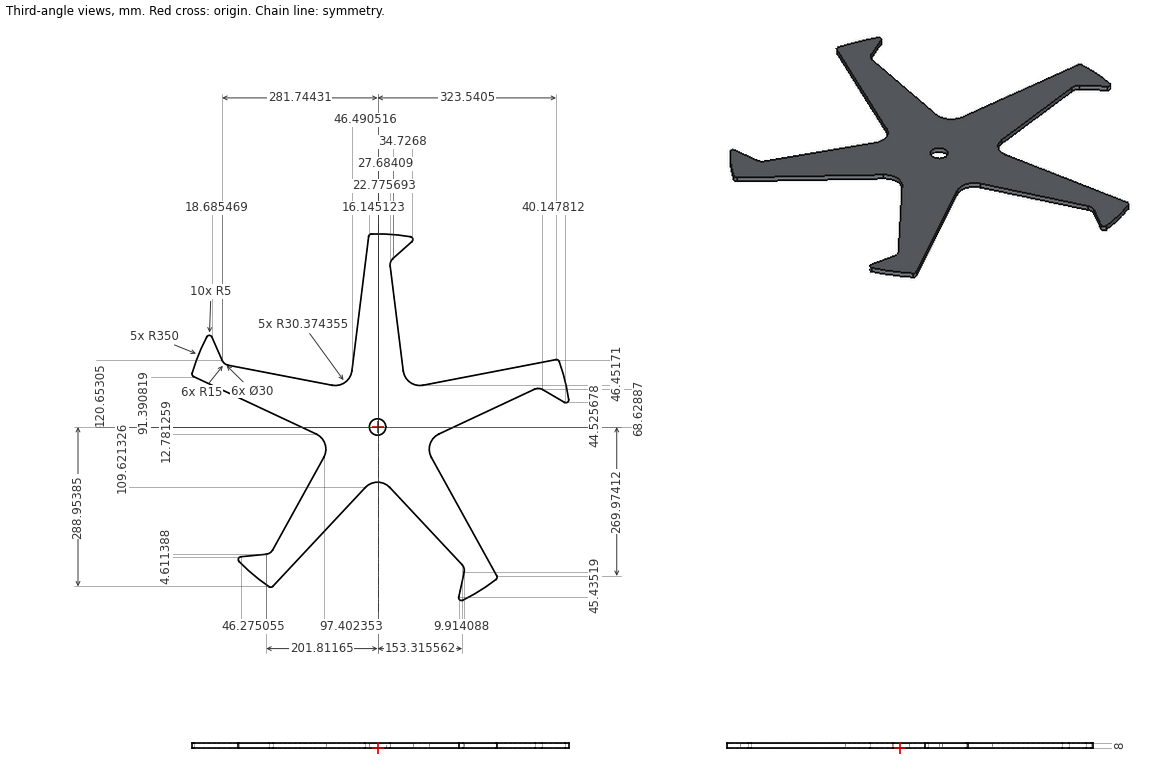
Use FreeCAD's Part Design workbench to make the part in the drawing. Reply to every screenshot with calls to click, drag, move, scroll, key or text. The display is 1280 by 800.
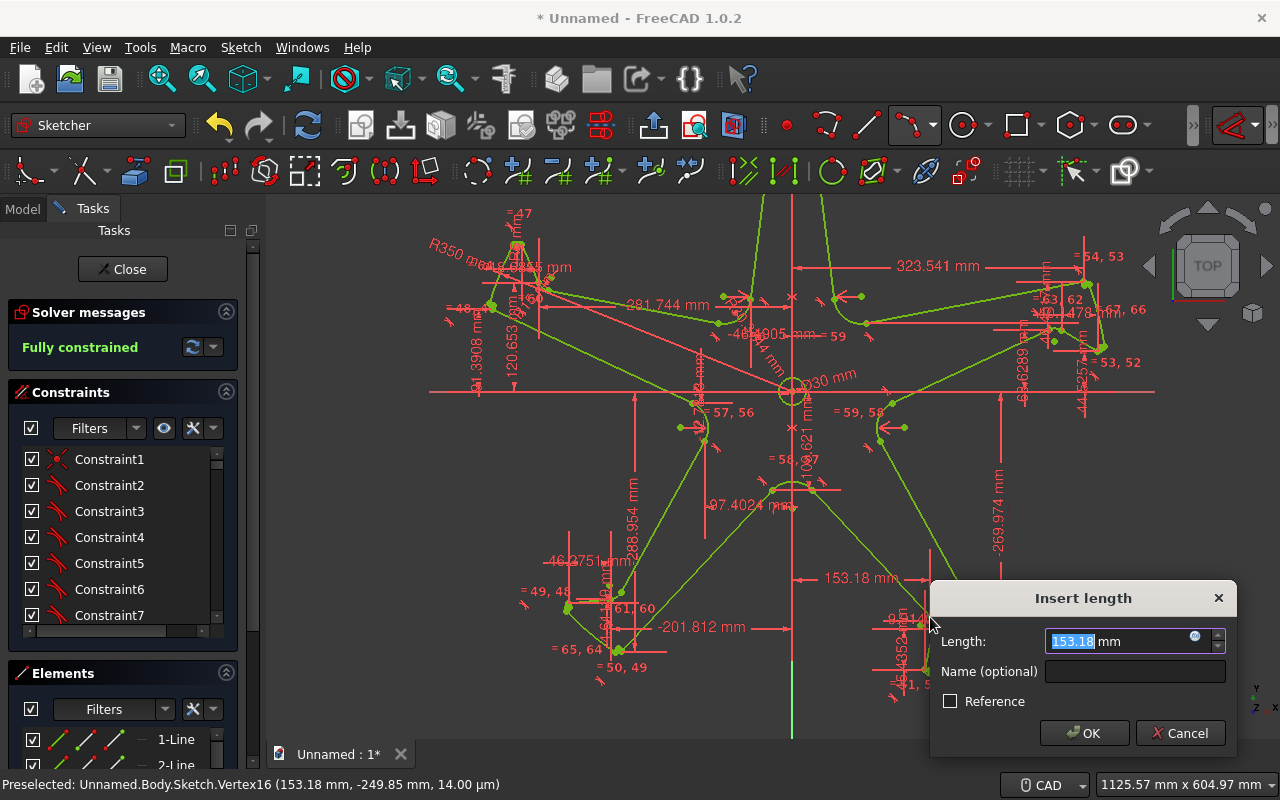
text(153.315562)
key(Return)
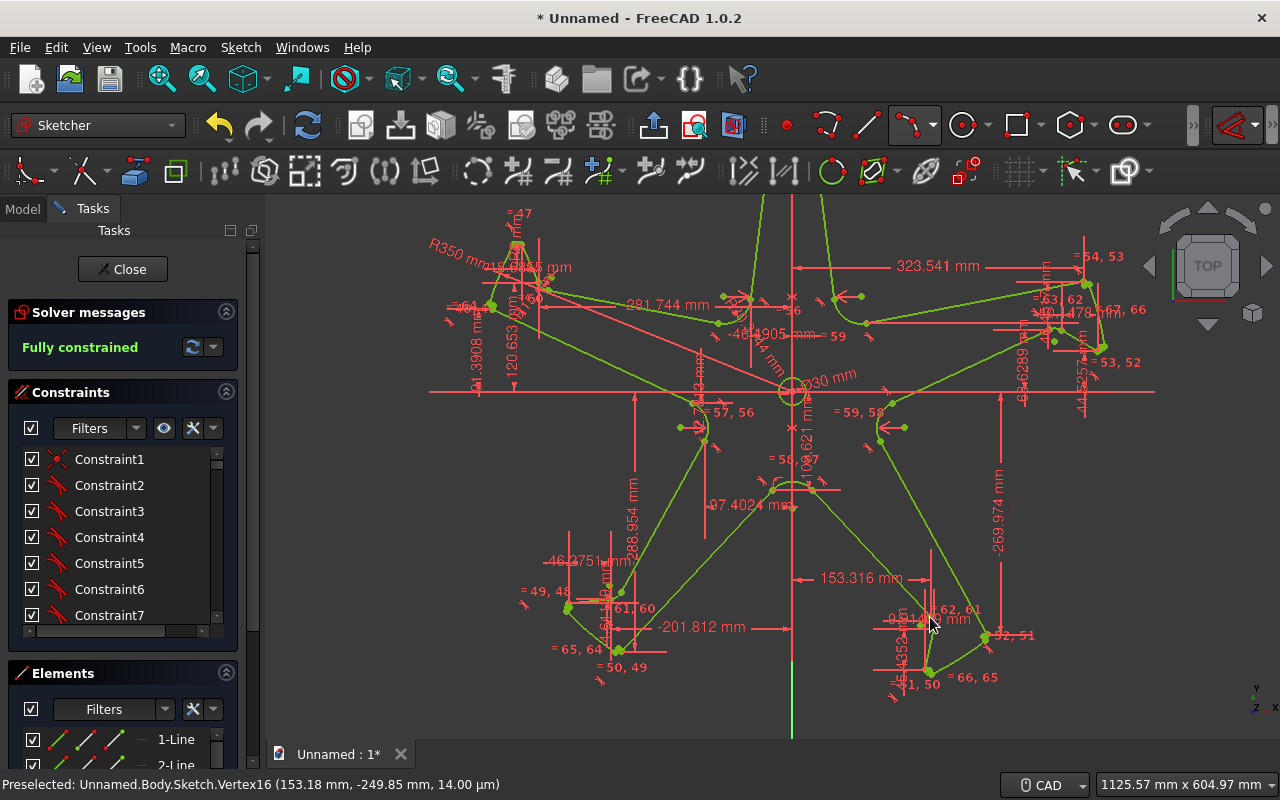
click(123, 269)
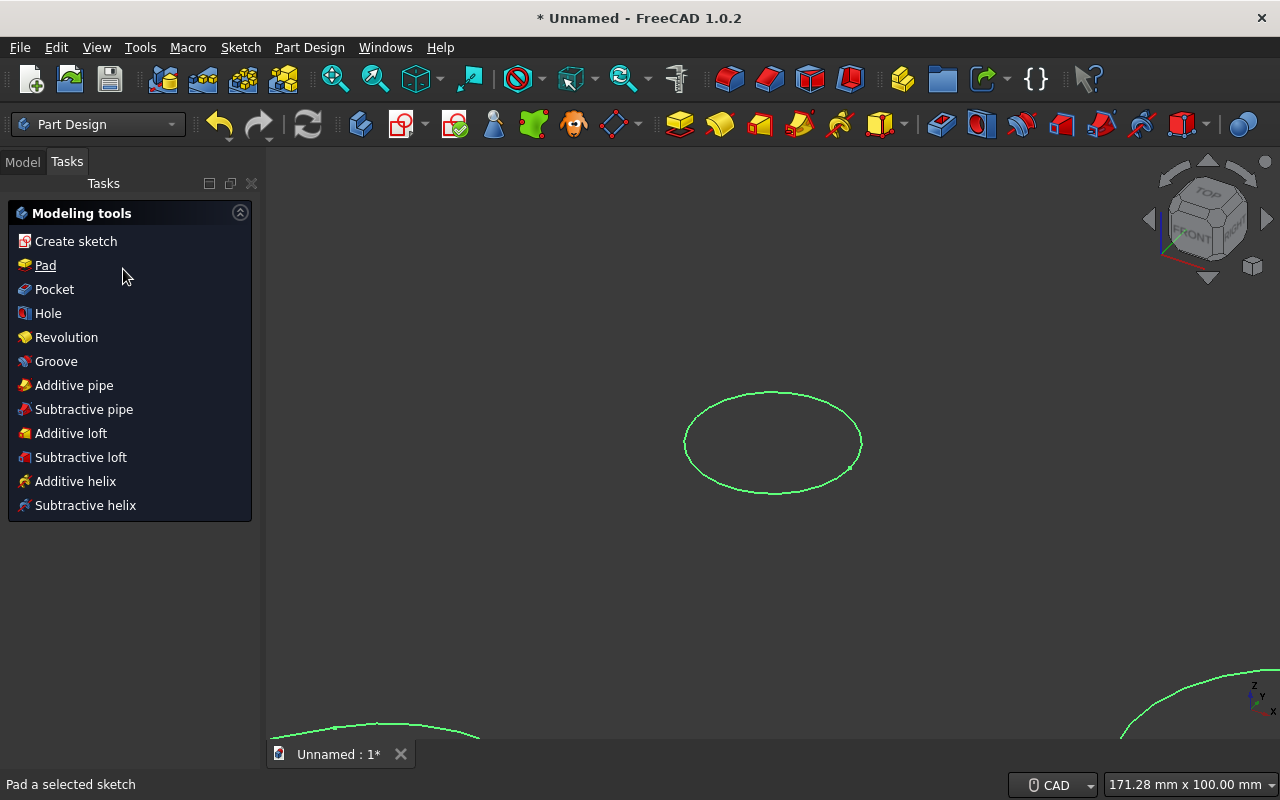
click(680, 124)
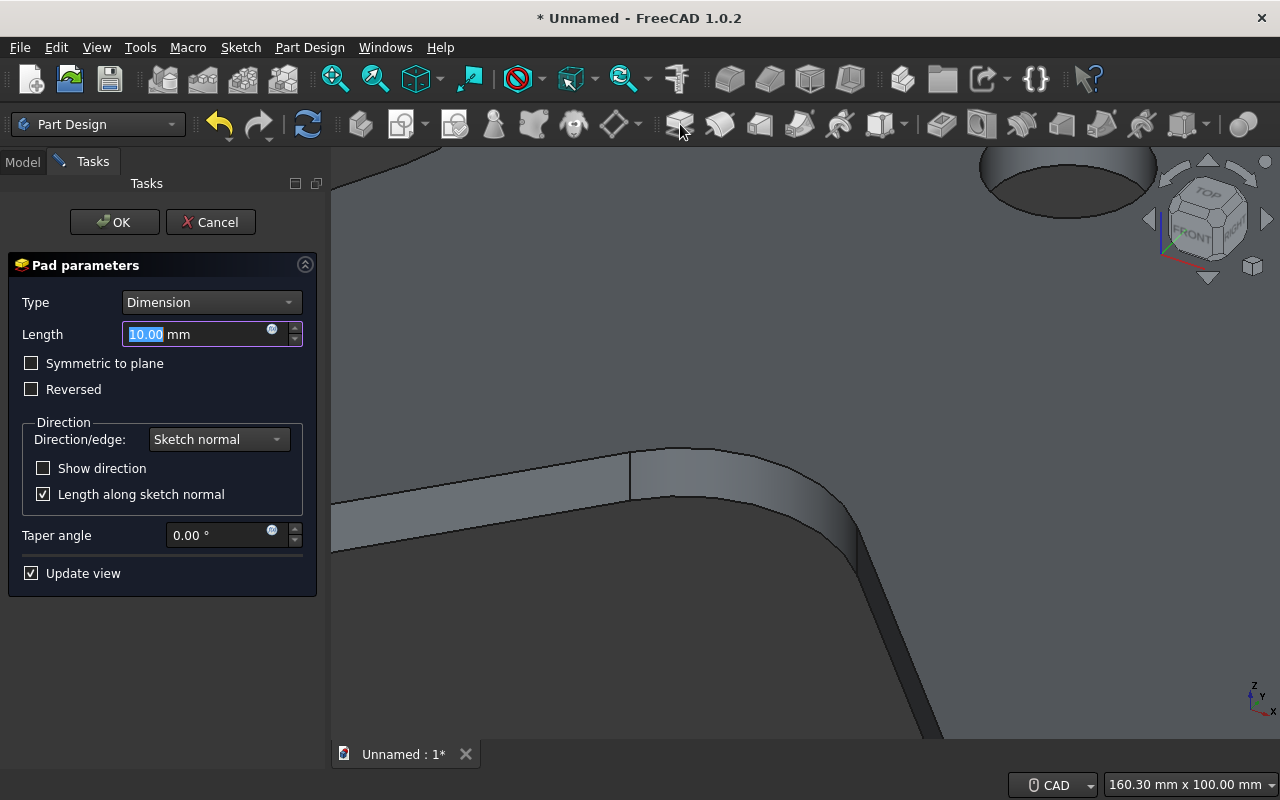
text(8)
key(Tab)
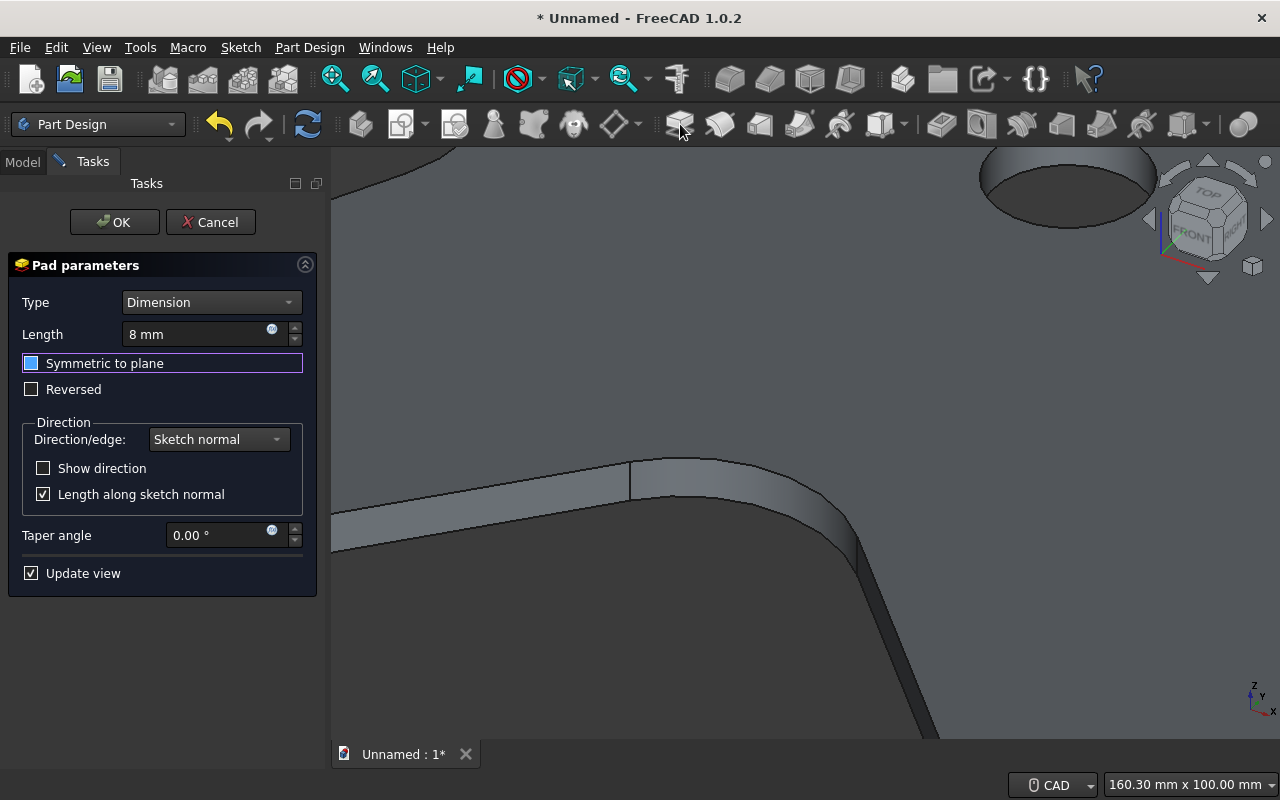
click(115, 222)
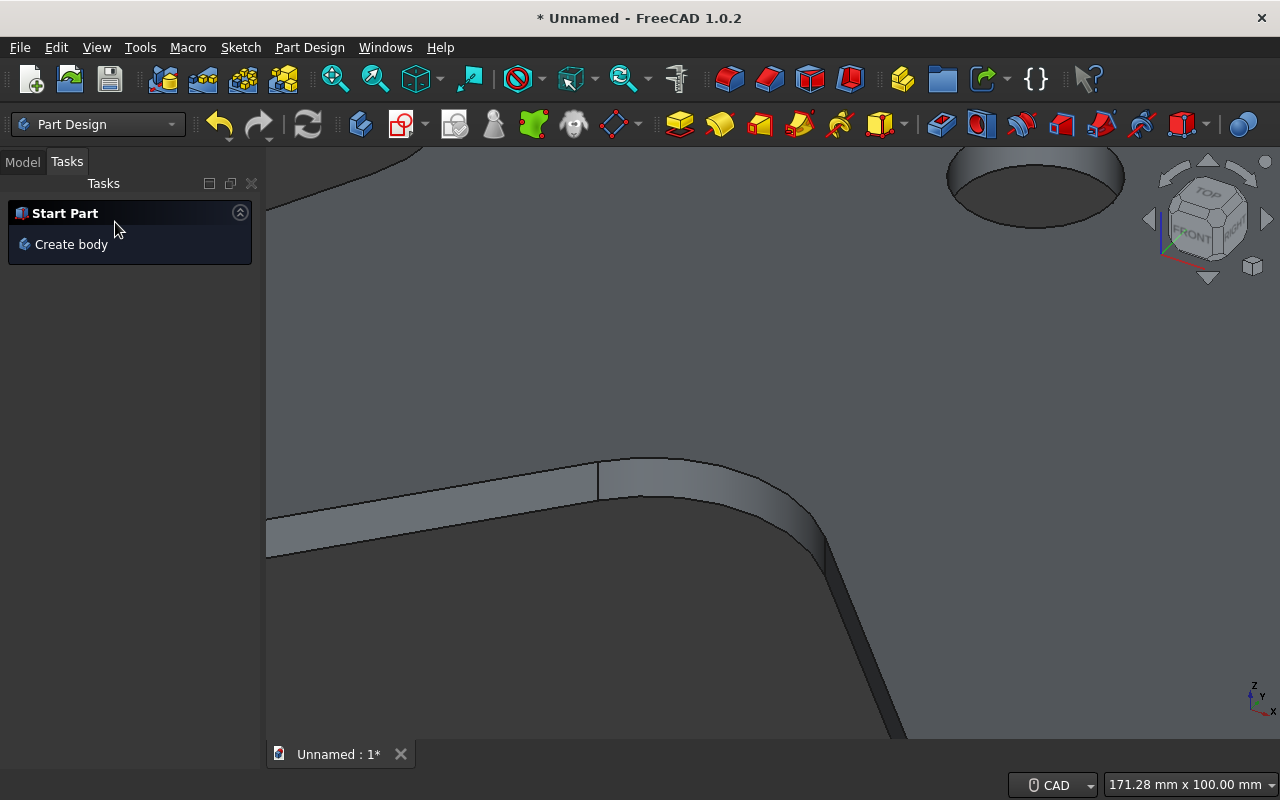
key(0)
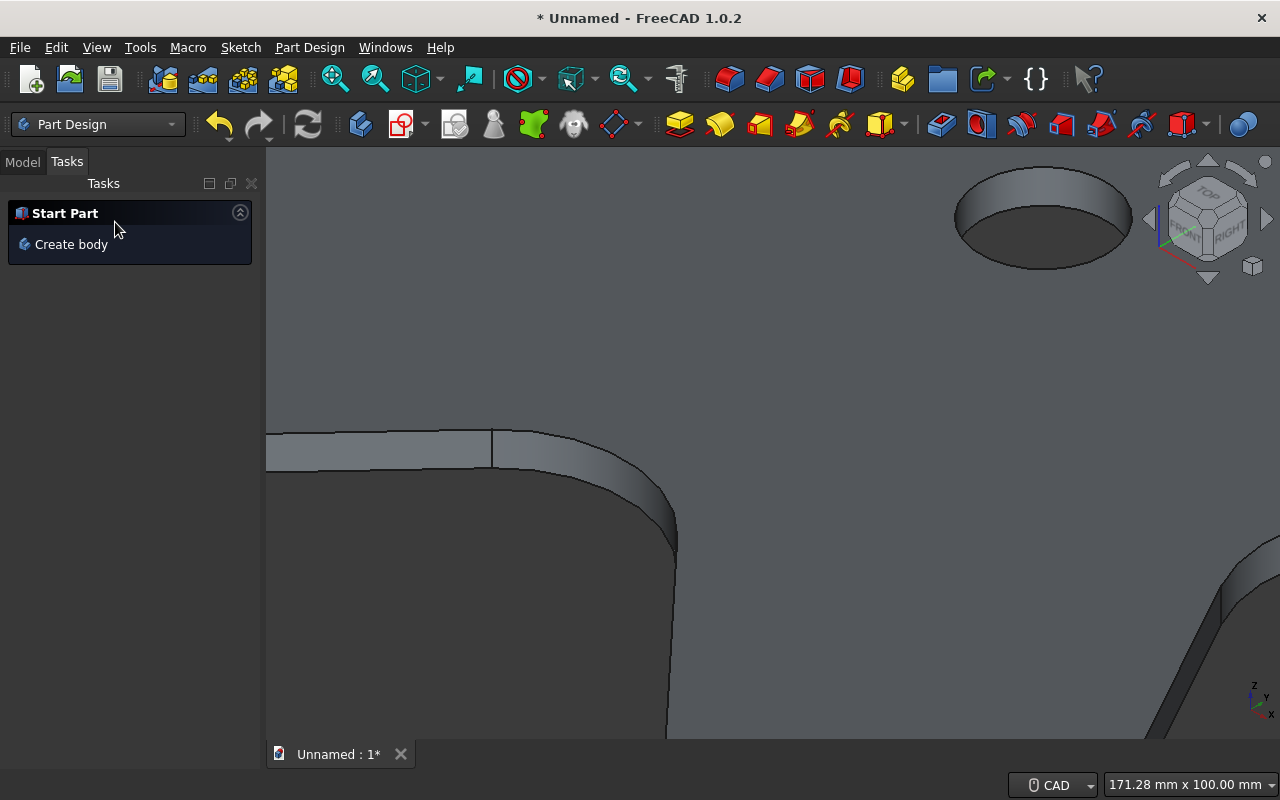
click(336, 80)